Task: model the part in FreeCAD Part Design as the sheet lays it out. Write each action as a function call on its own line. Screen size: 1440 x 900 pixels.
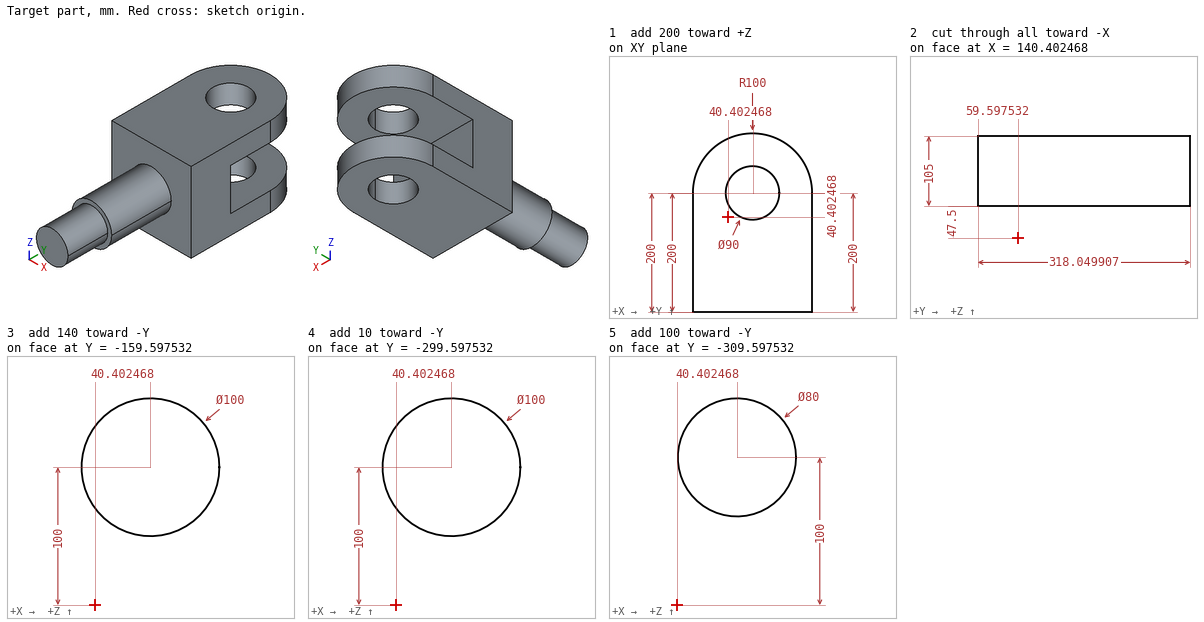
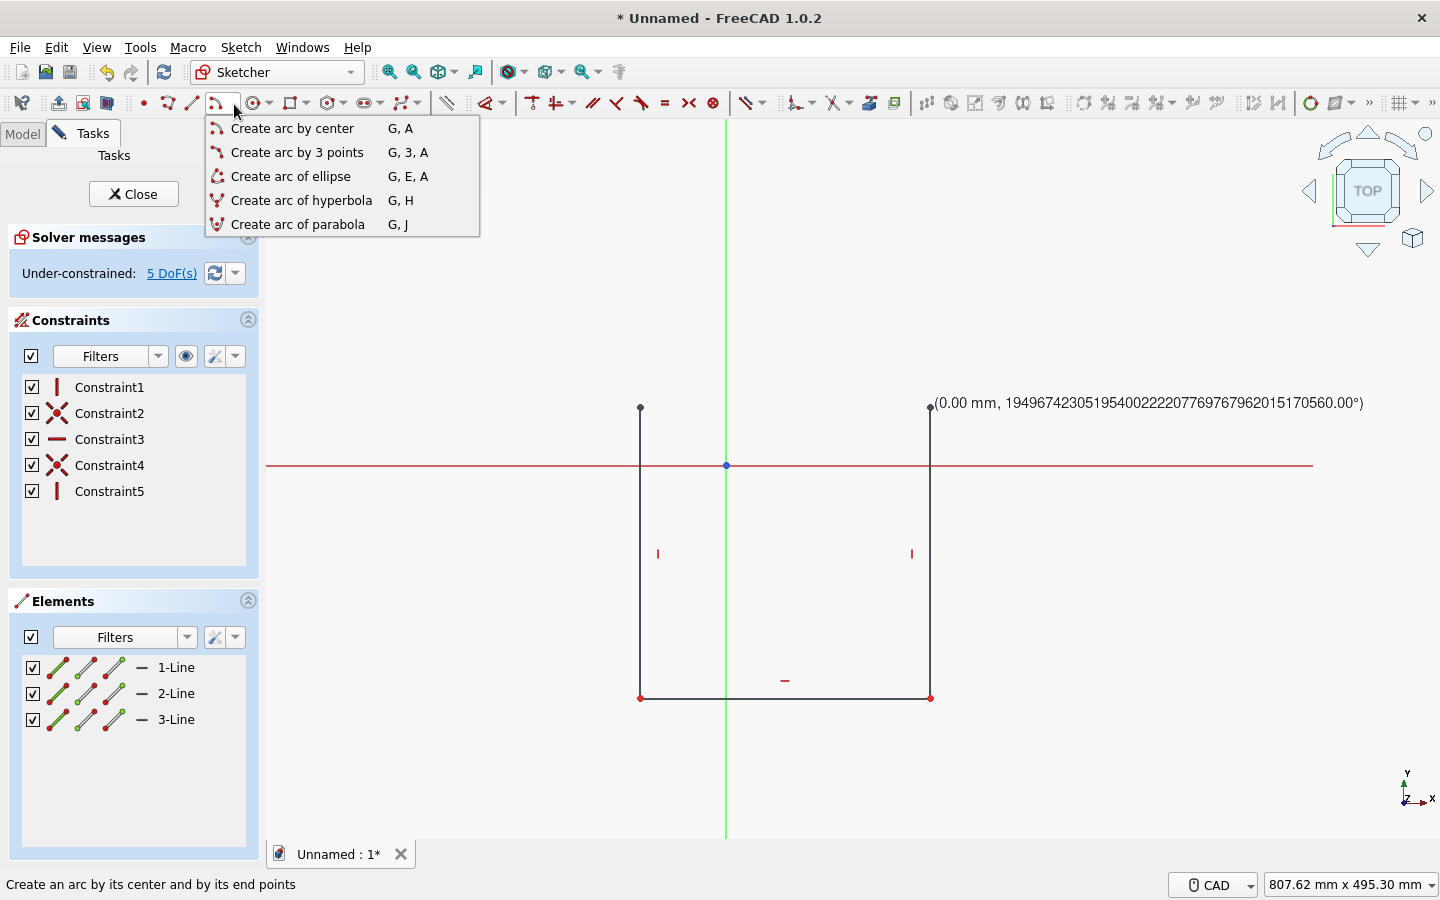
click(342, 152)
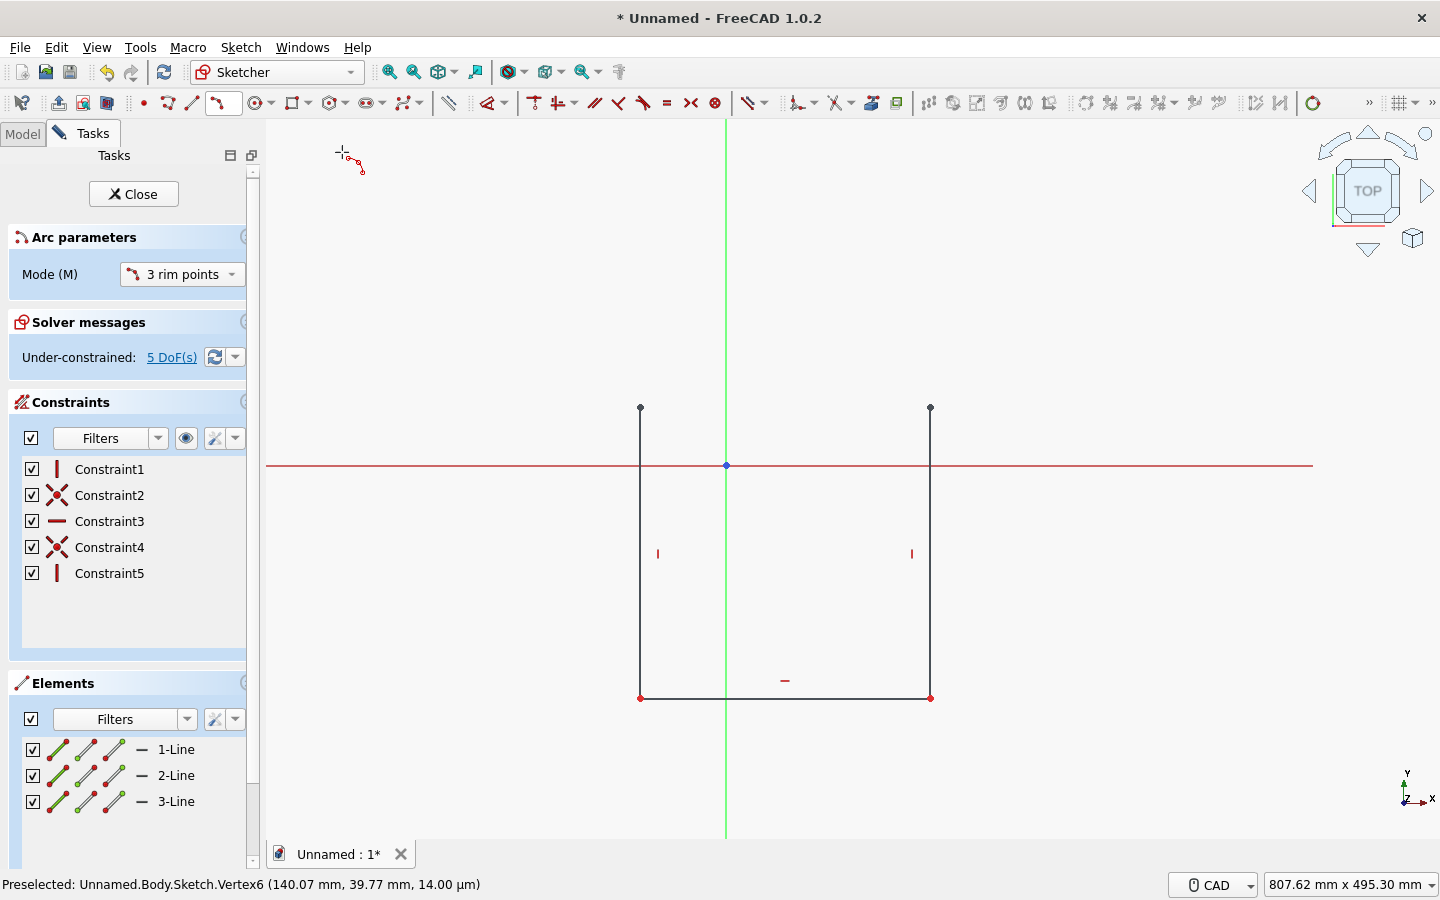
click(930, 408)
click(640, 408)
click(785, 262)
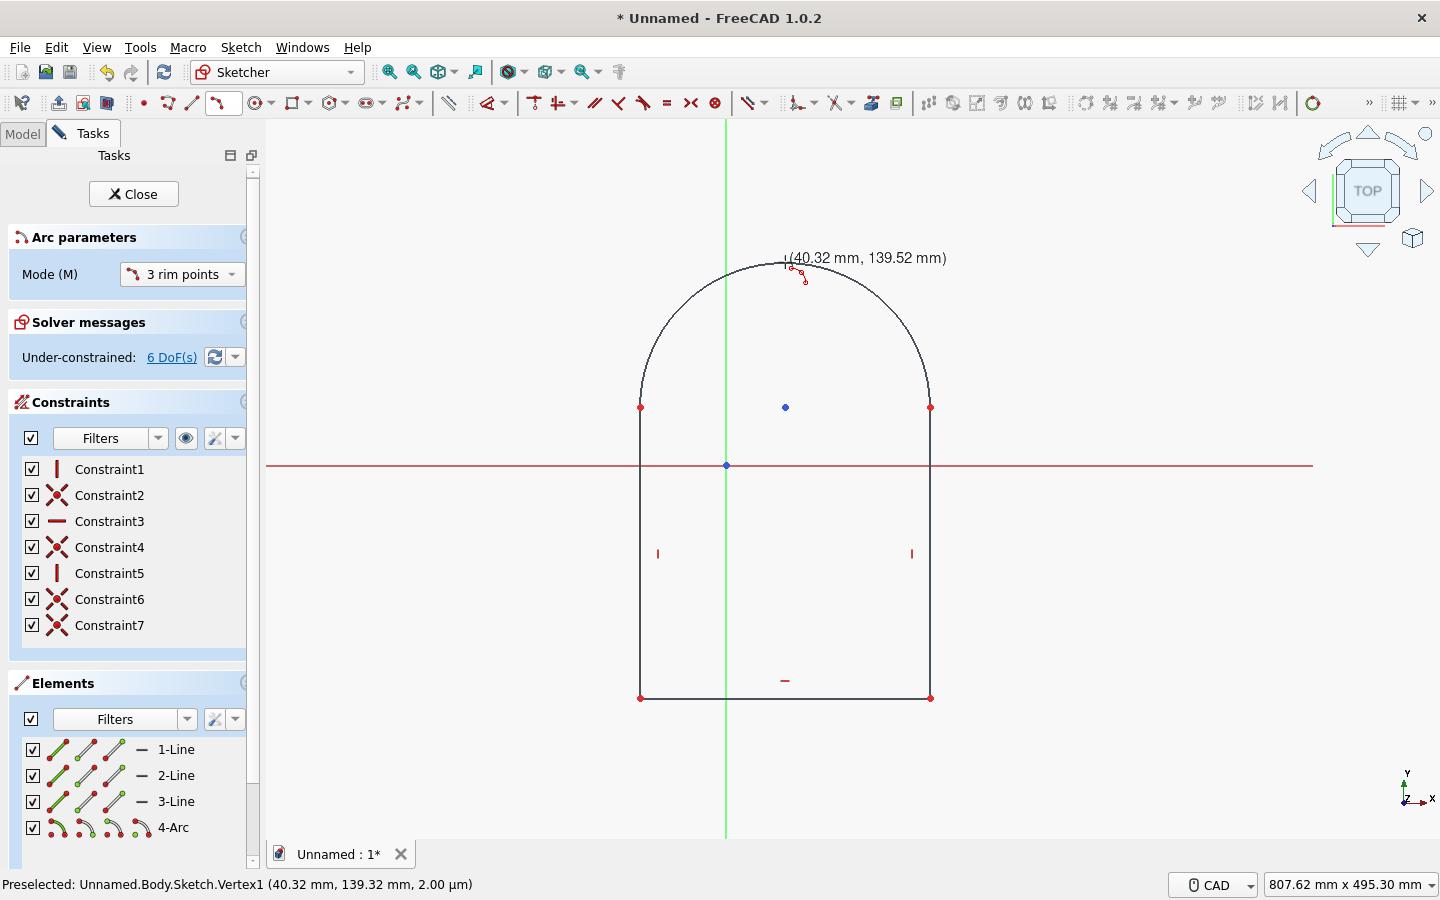
click(256, 104)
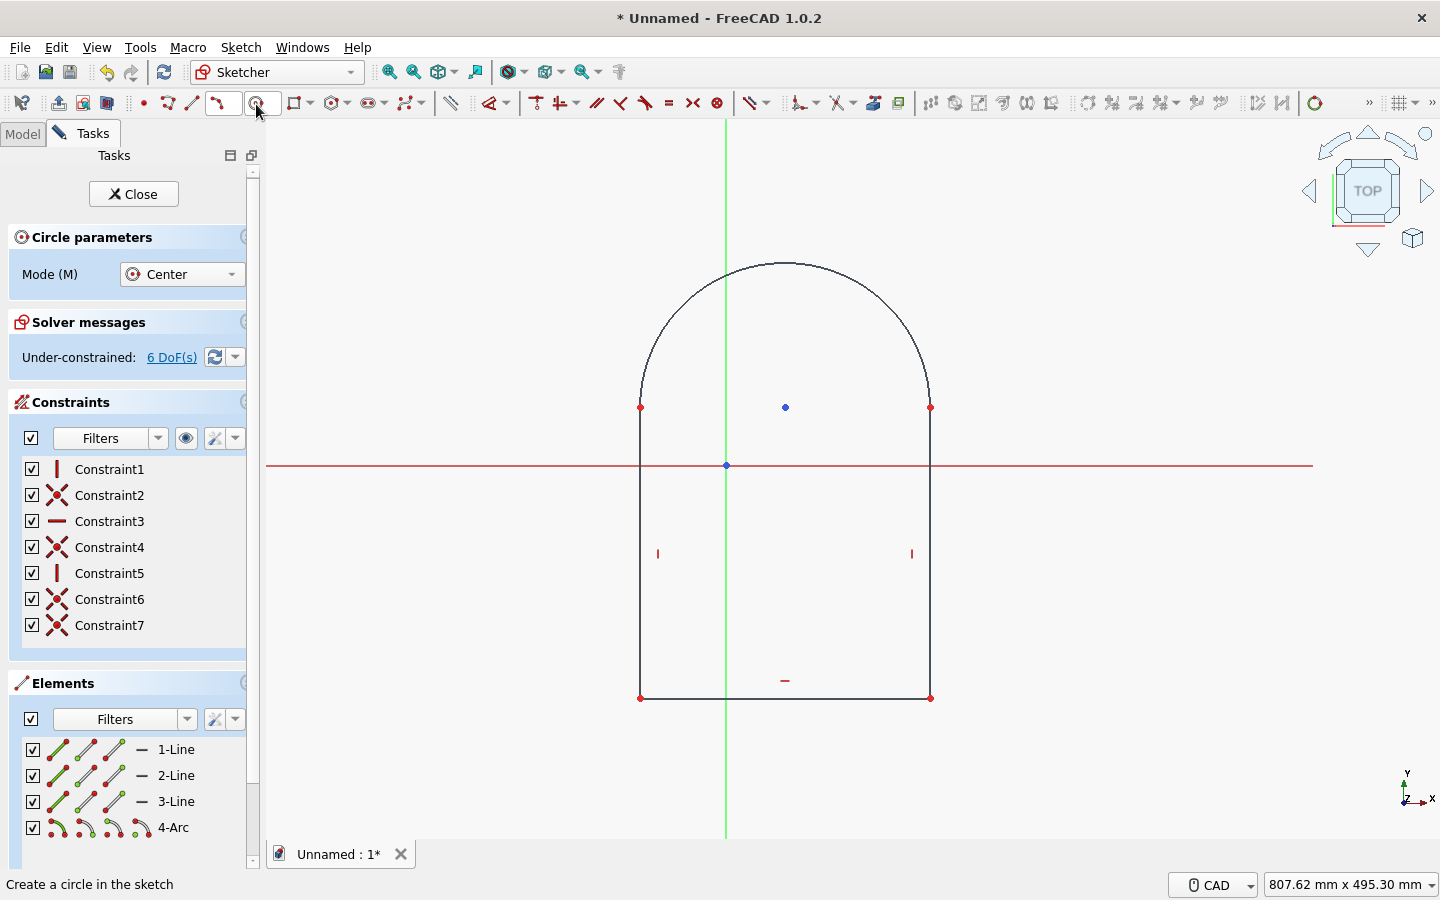
click(785, 407)
click(831, 361)
key(Escape)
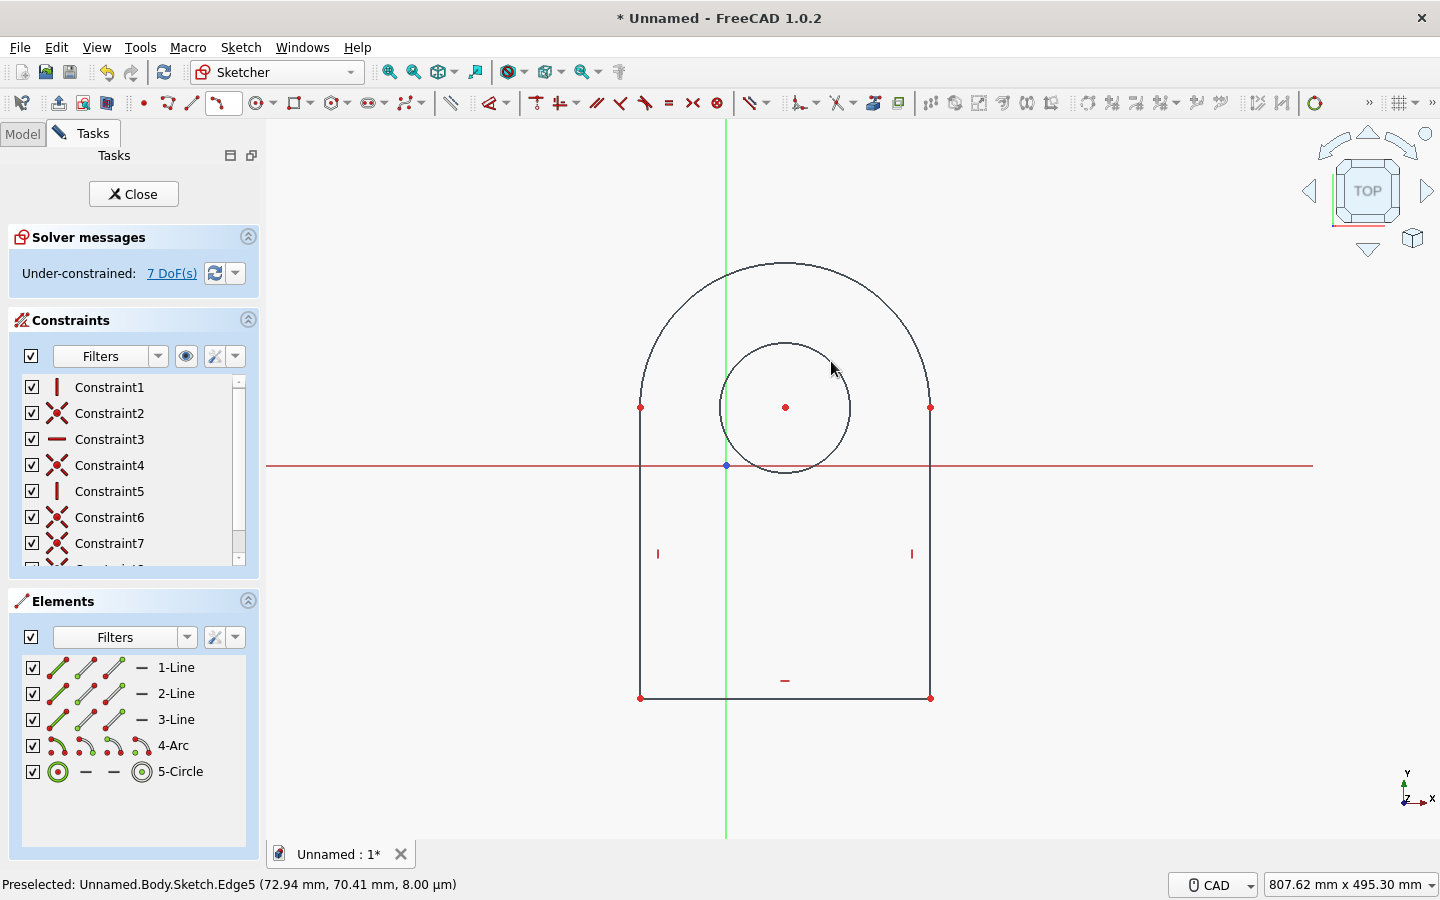
click(490, 104)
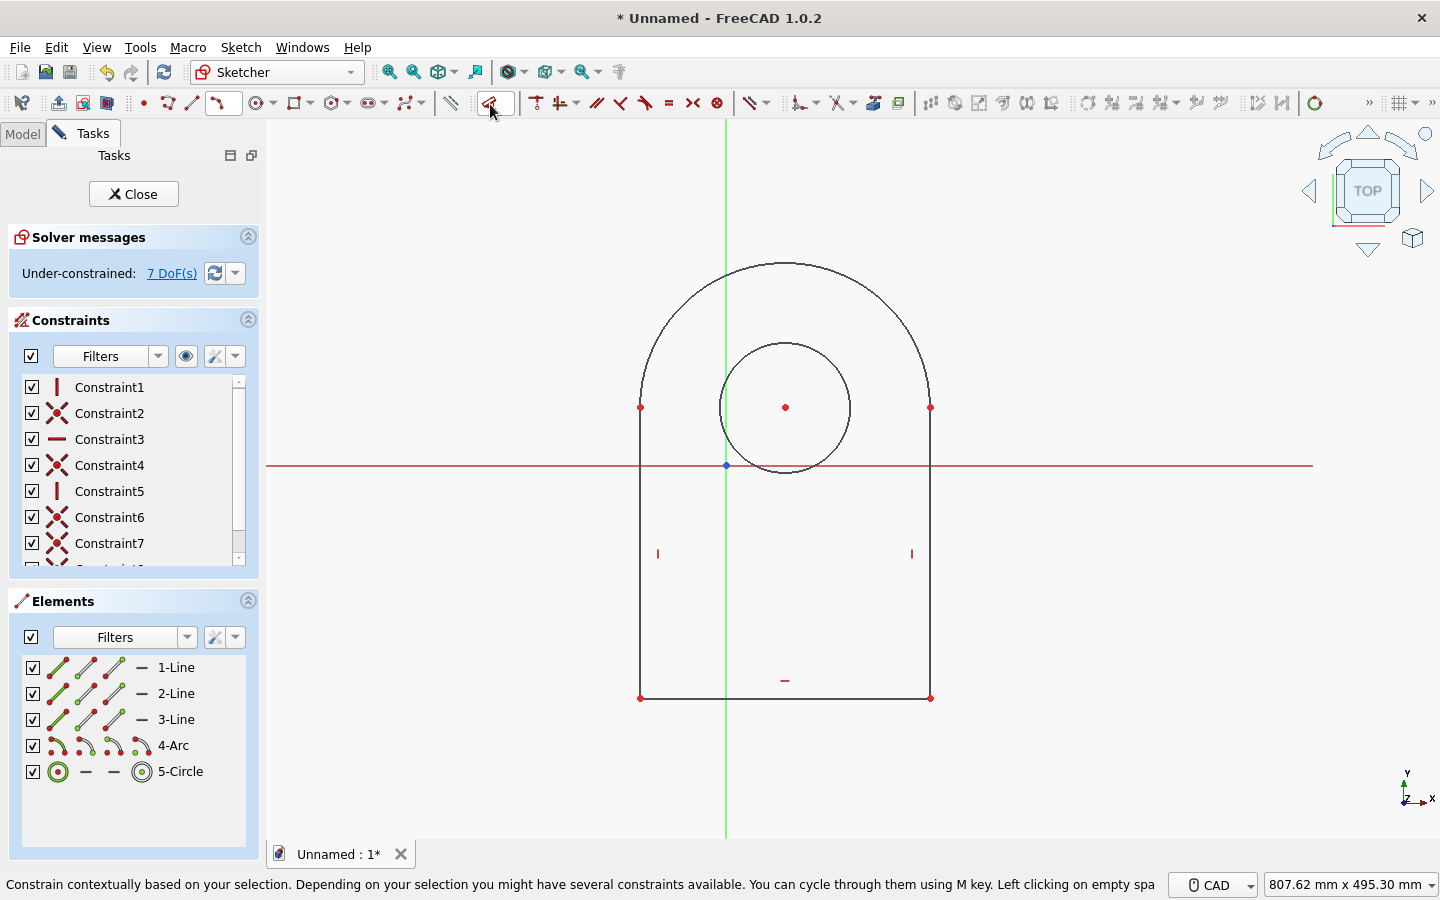
click(870, 291)
click(889, 265)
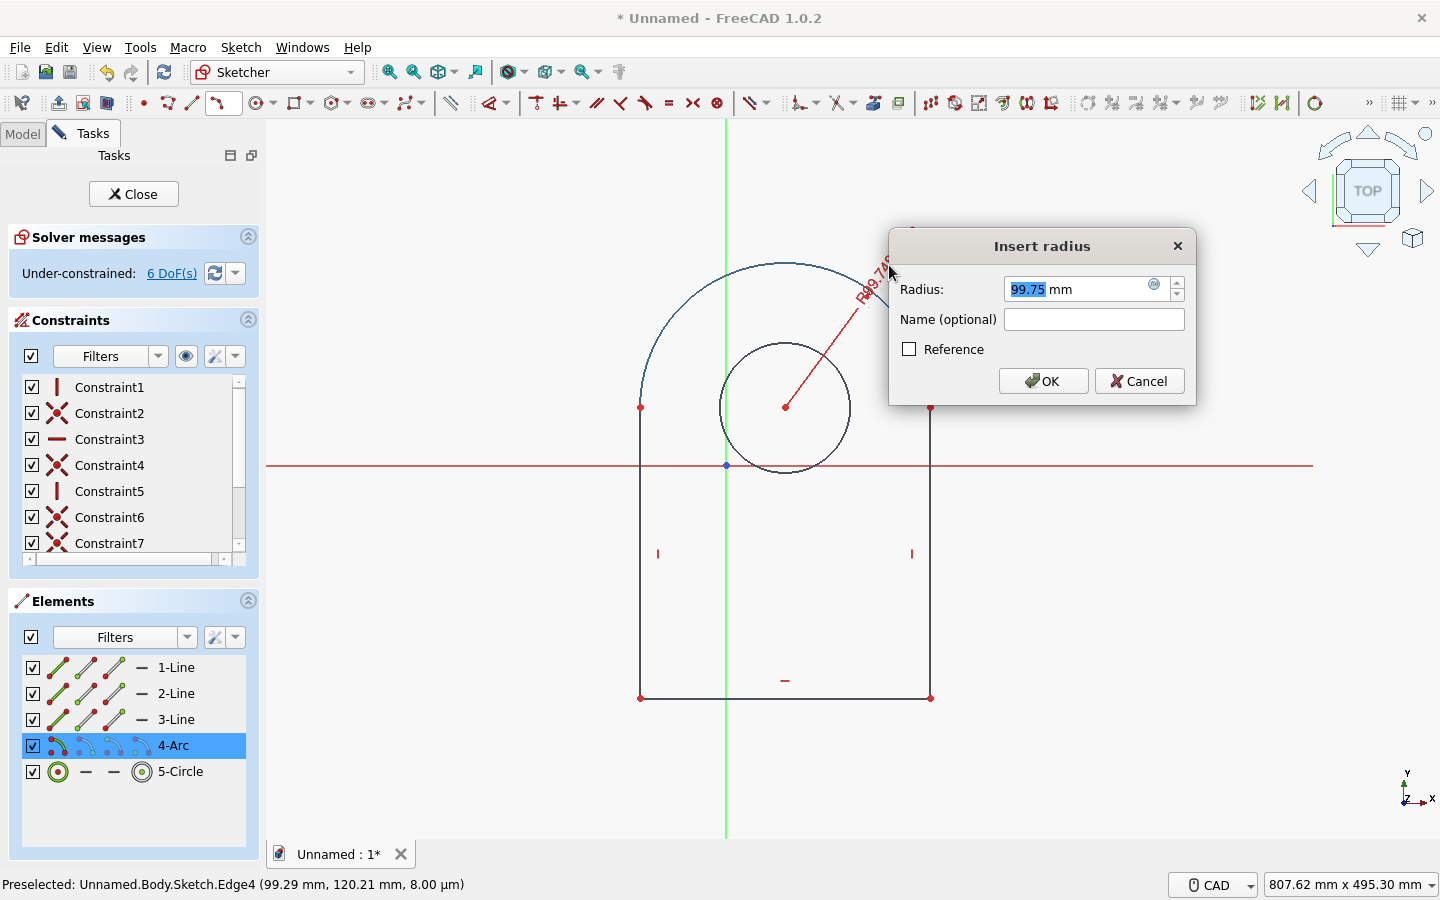
text(100)
key(Return)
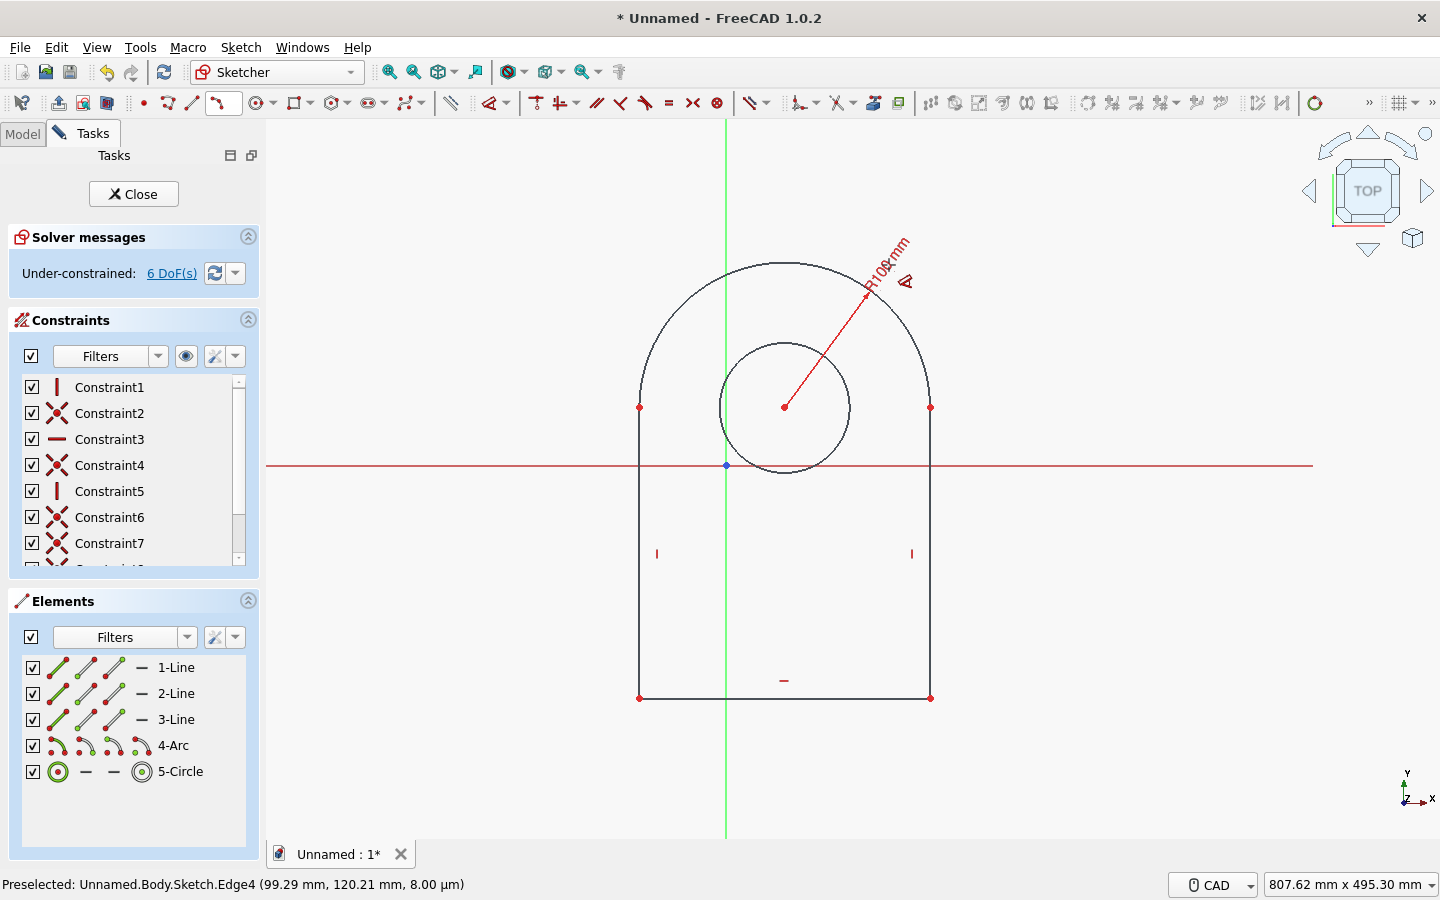
click(831, 362)
click(854, 339)